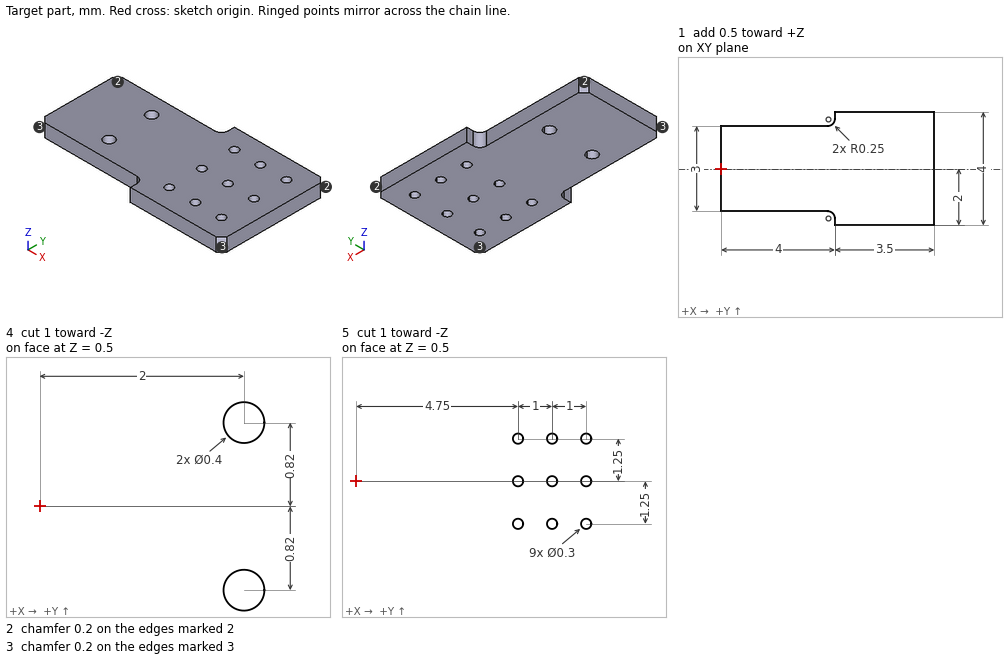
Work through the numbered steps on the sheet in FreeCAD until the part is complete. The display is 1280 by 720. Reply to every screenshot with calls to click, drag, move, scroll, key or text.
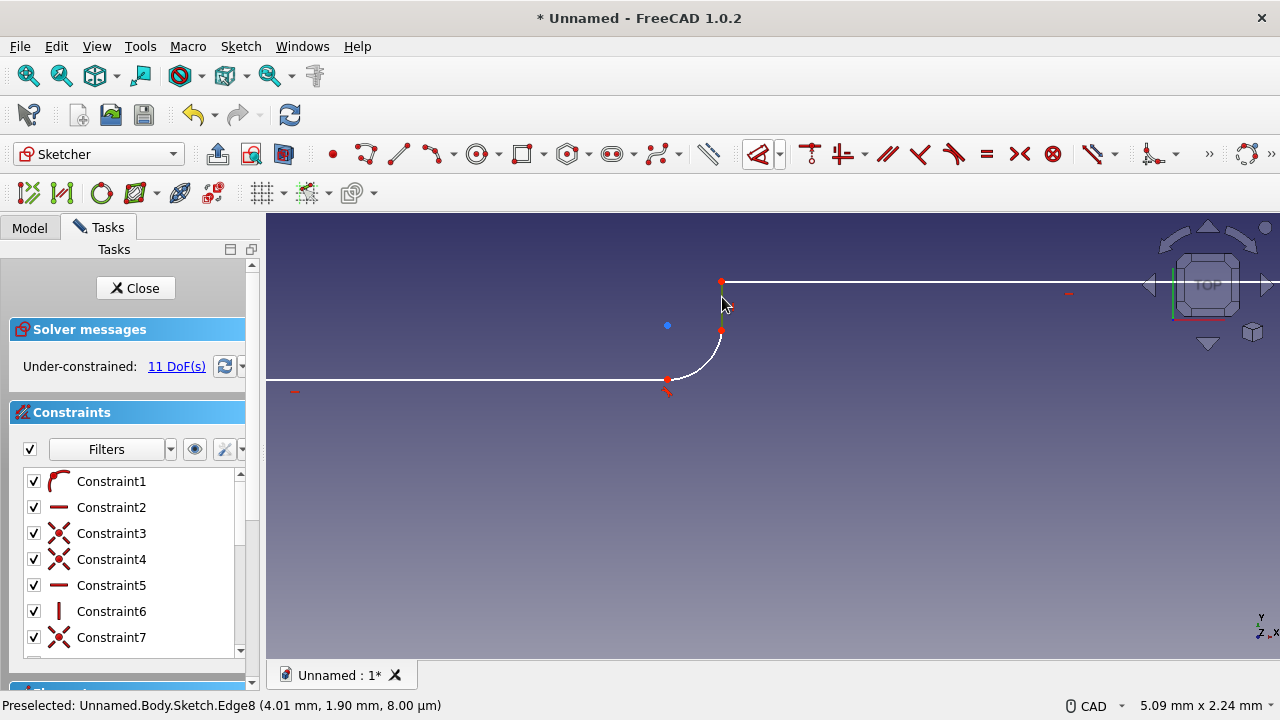
click(691, 375)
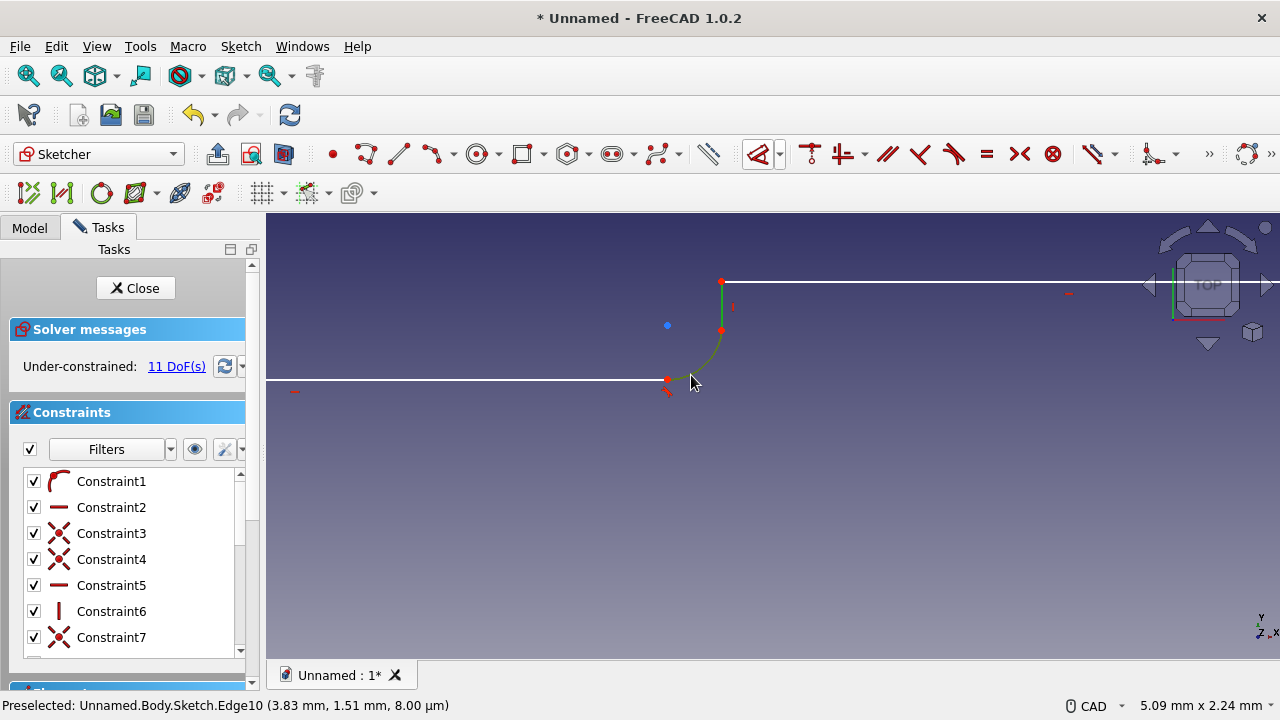
key(t)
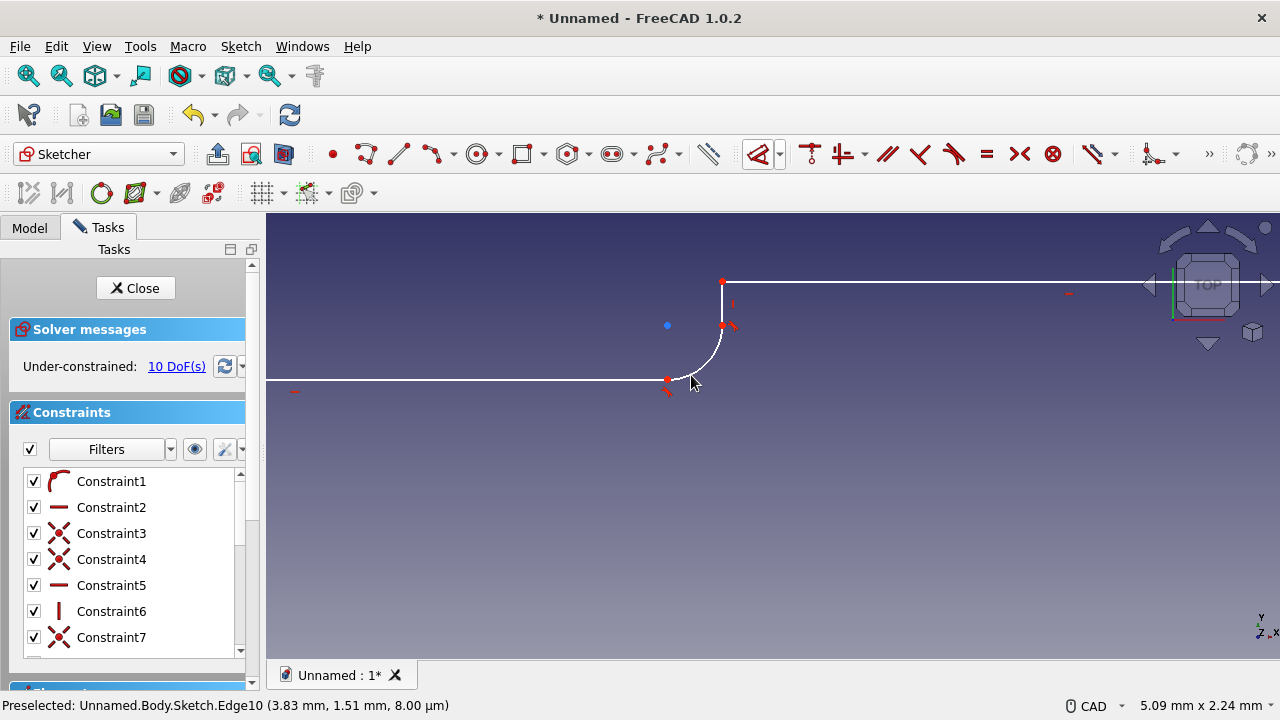
scroll(724, 296, down, 5)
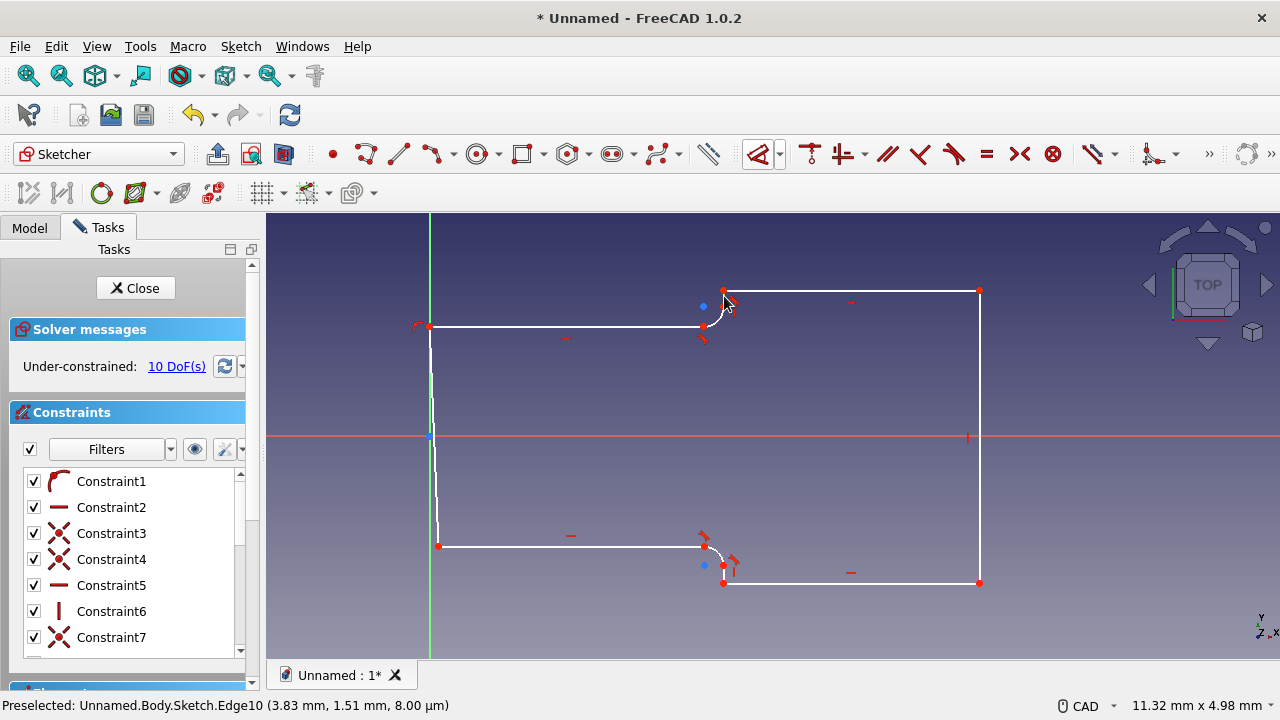
scroll(436, 481, up, 5)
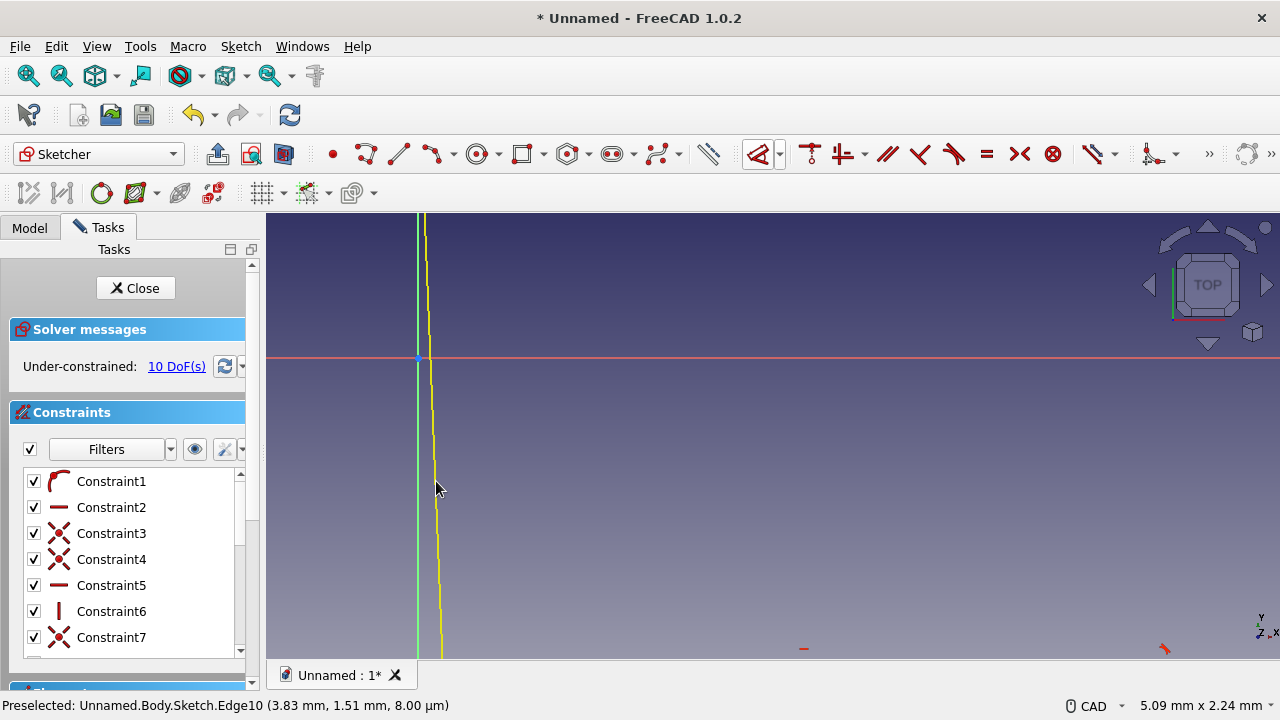
click(435, 480)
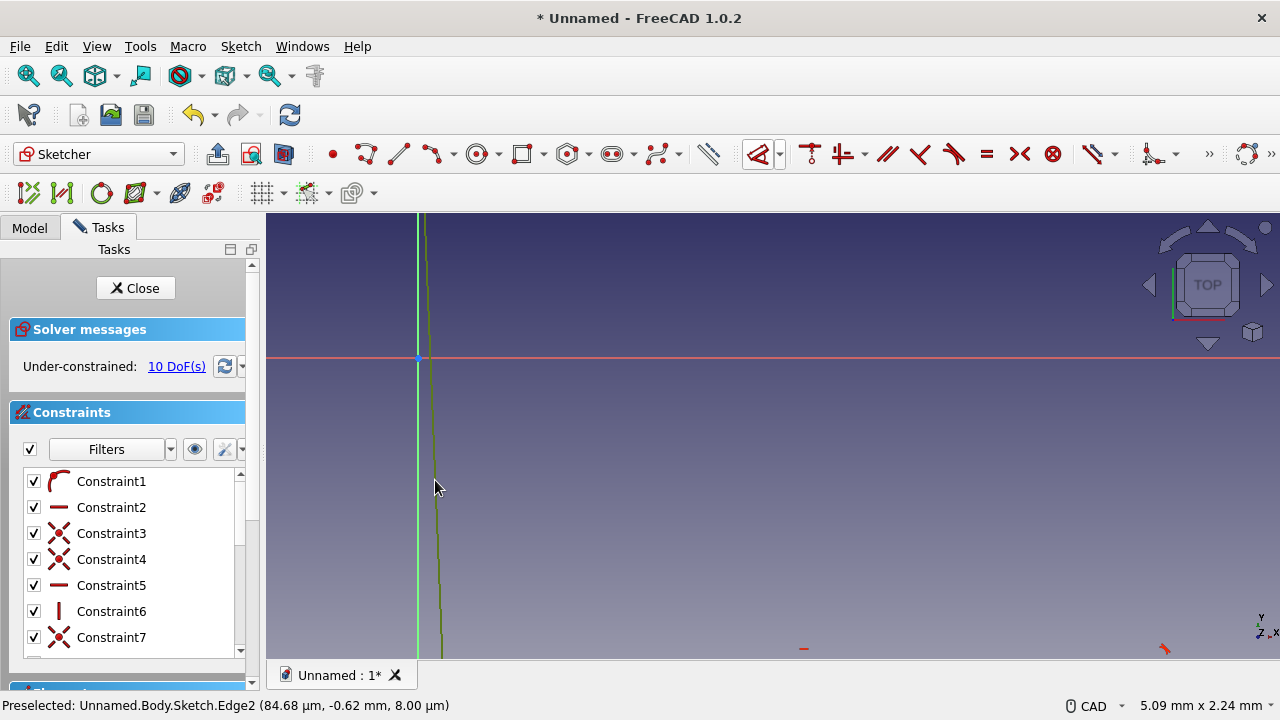
click(864, 154)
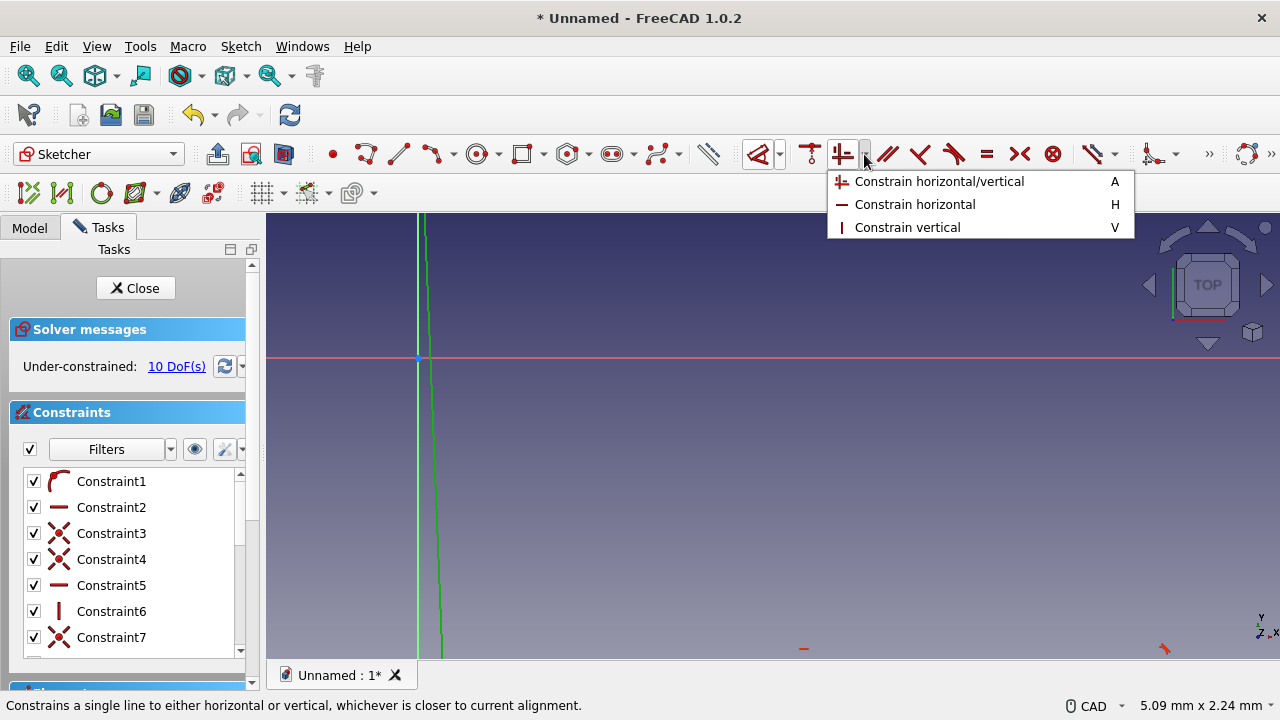
click(981, 228)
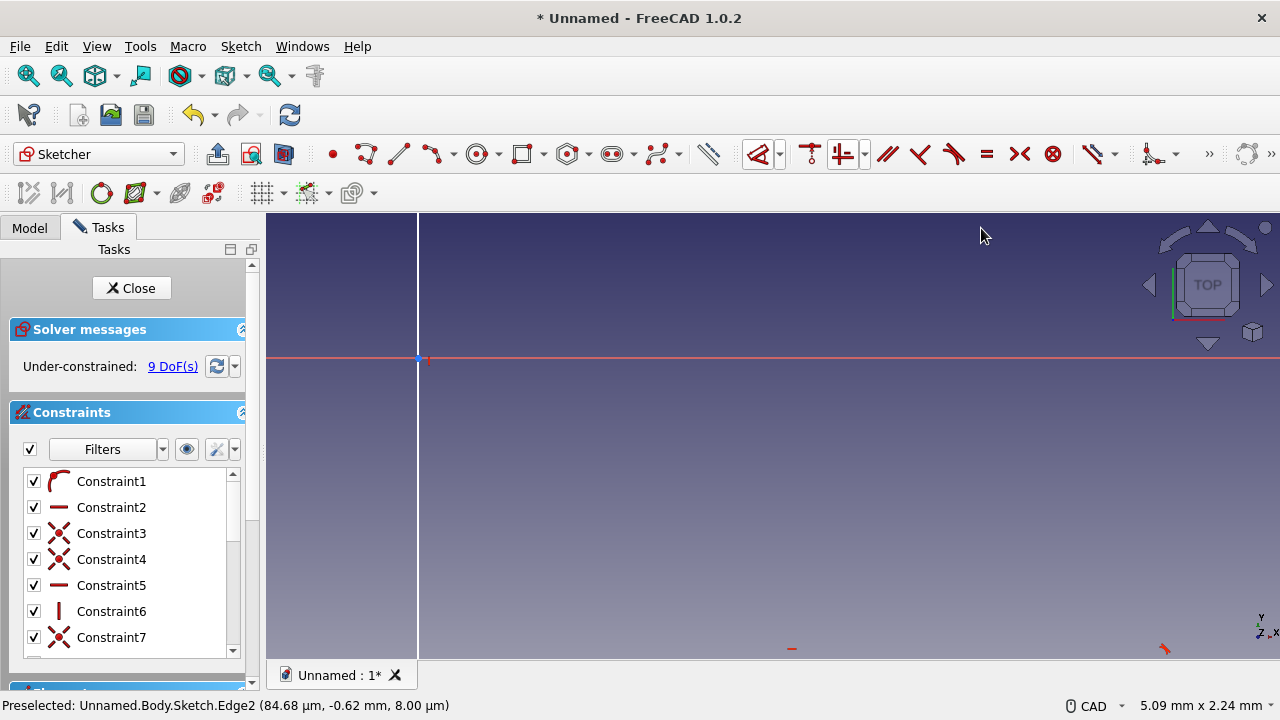
scroll(436, 481, down, 5)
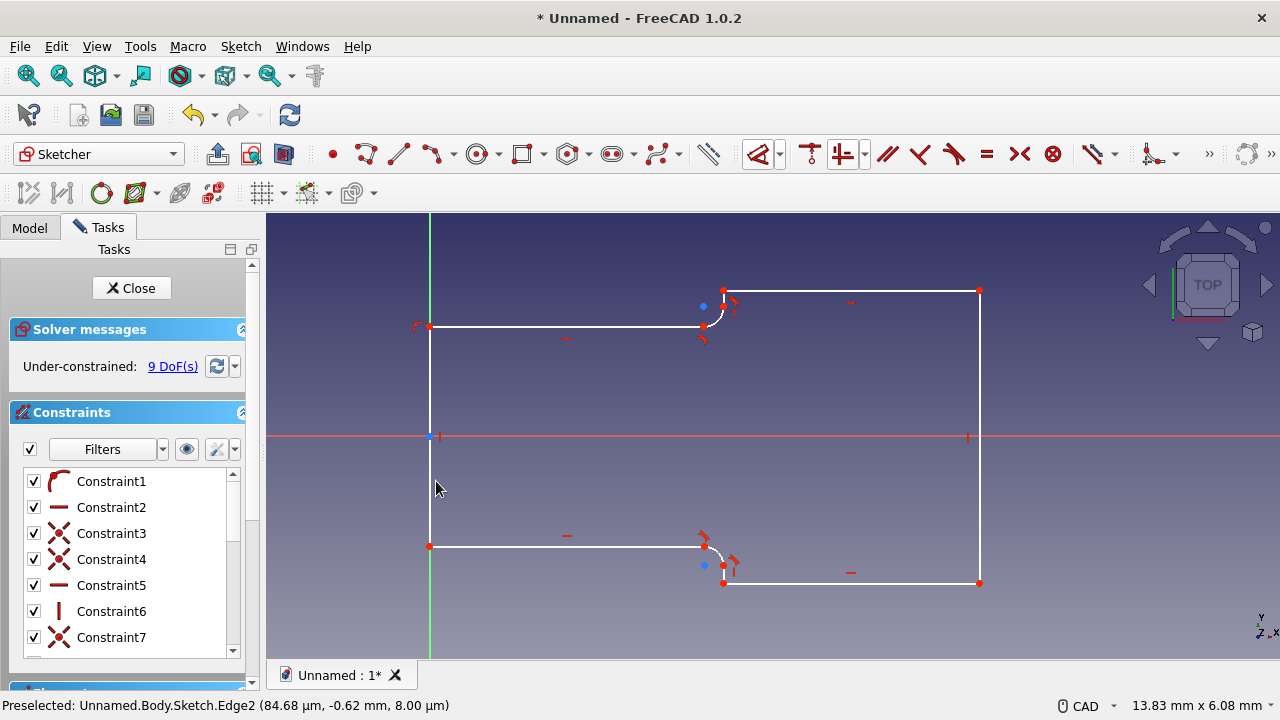
scroll(721, 557, up, 3)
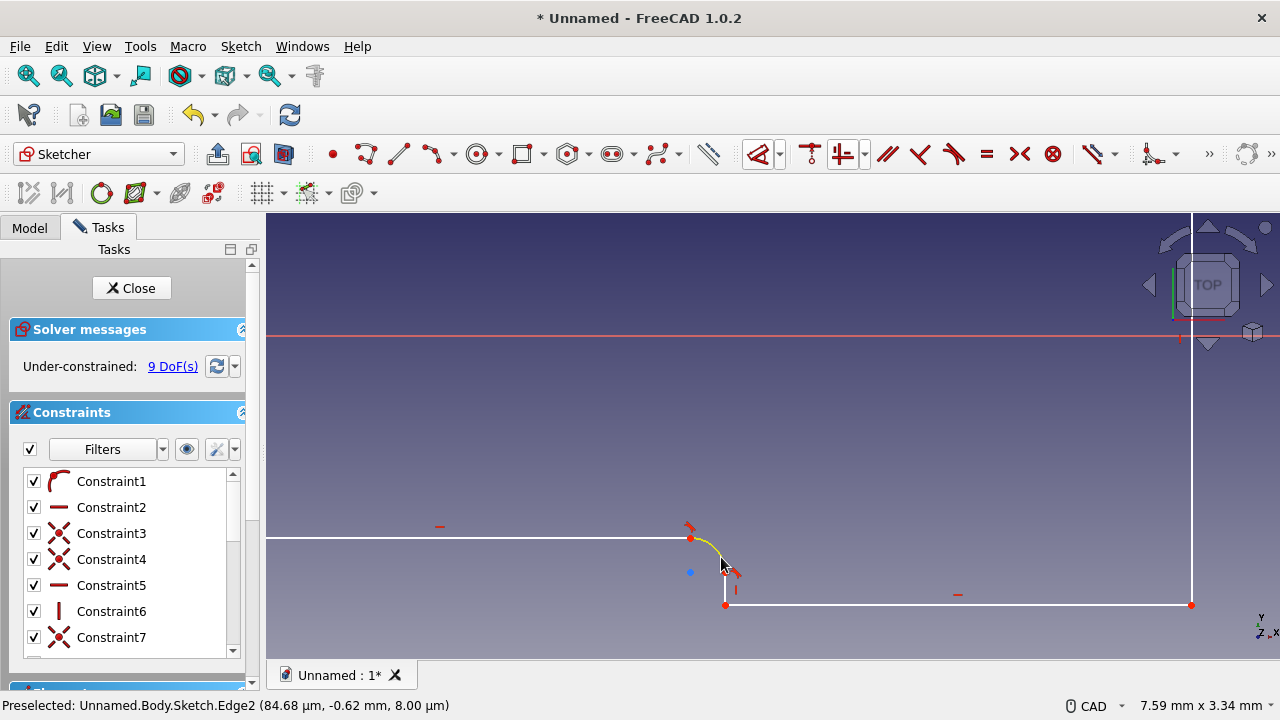
click(721, 557)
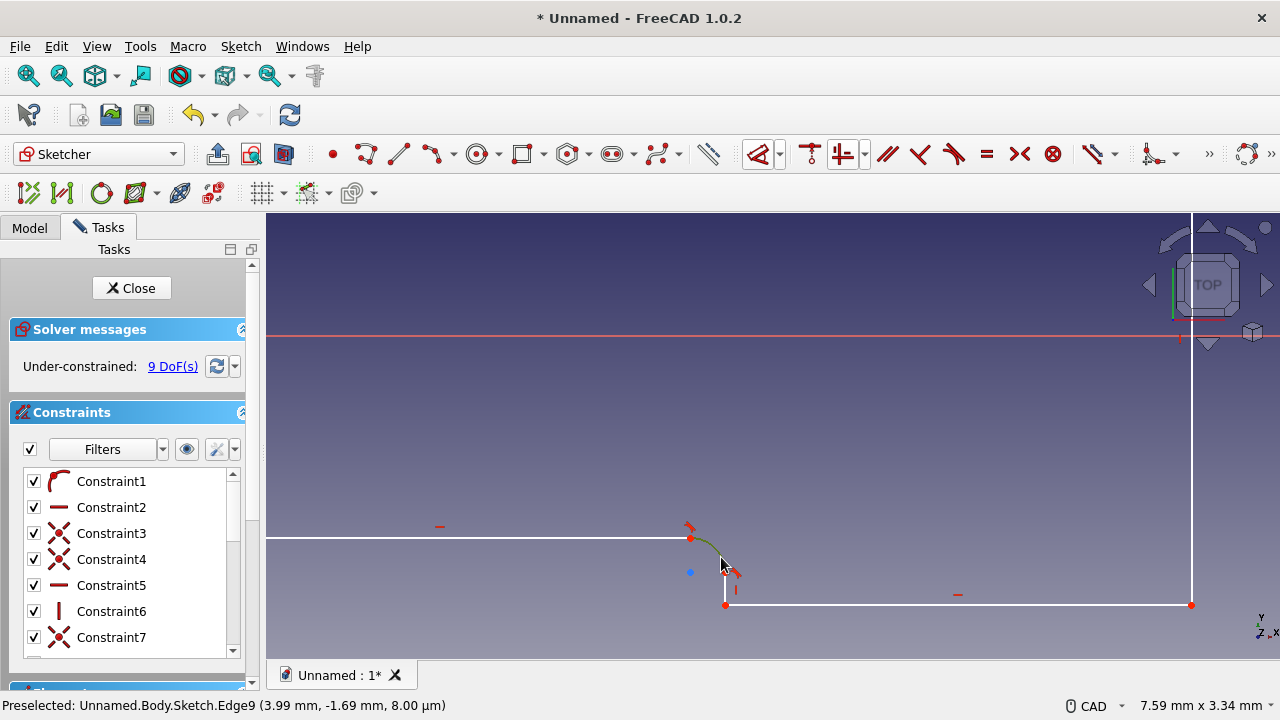
scroll(721, 557, down, 3)